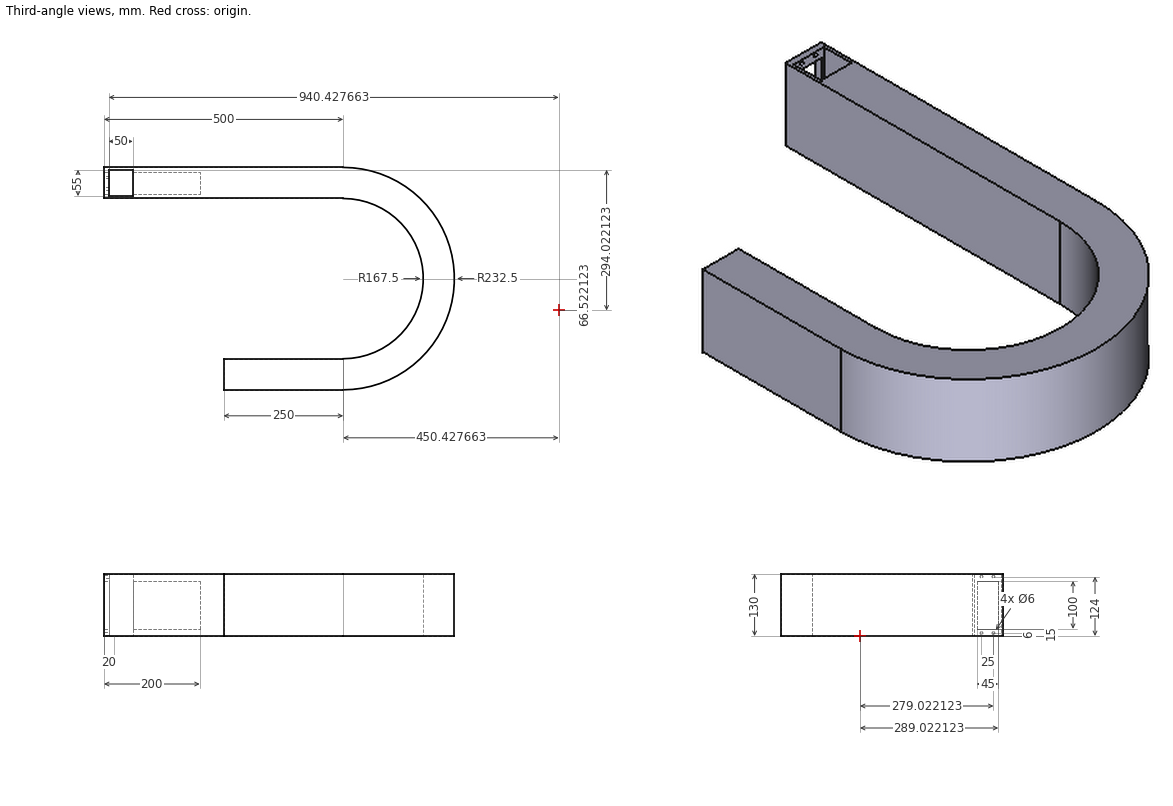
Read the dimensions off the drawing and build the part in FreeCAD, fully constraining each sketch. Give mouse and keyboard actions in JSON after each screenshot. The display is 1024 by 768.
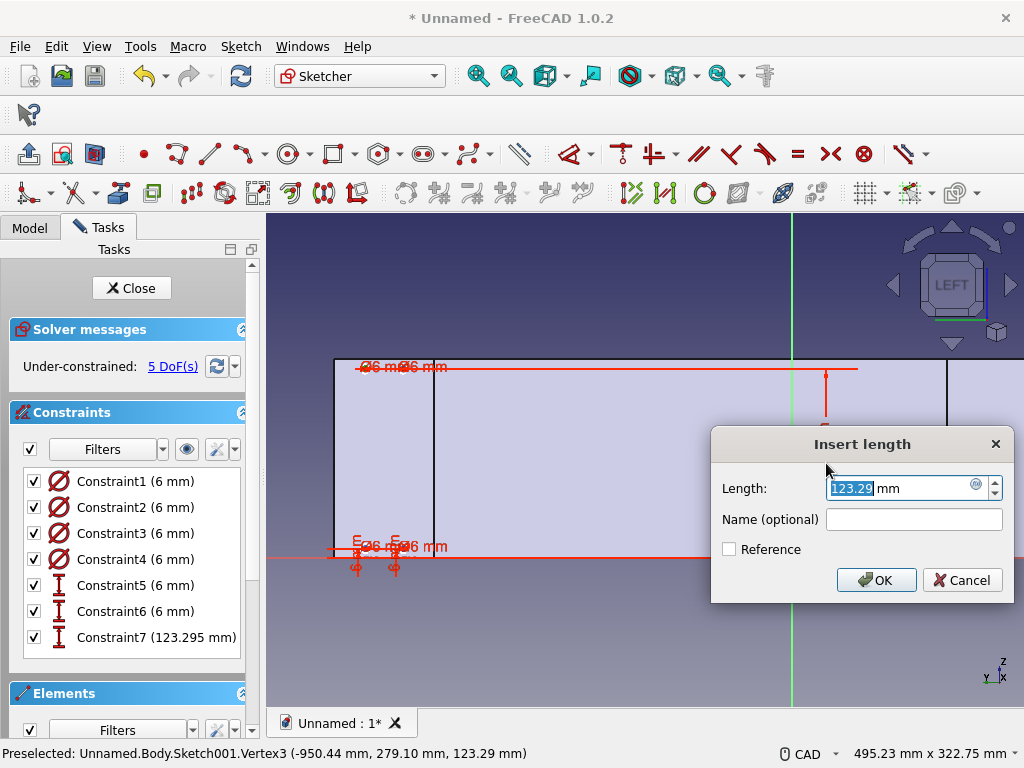
{"action": "type", "text": "124"}
{"action": "key", "text": "Return"}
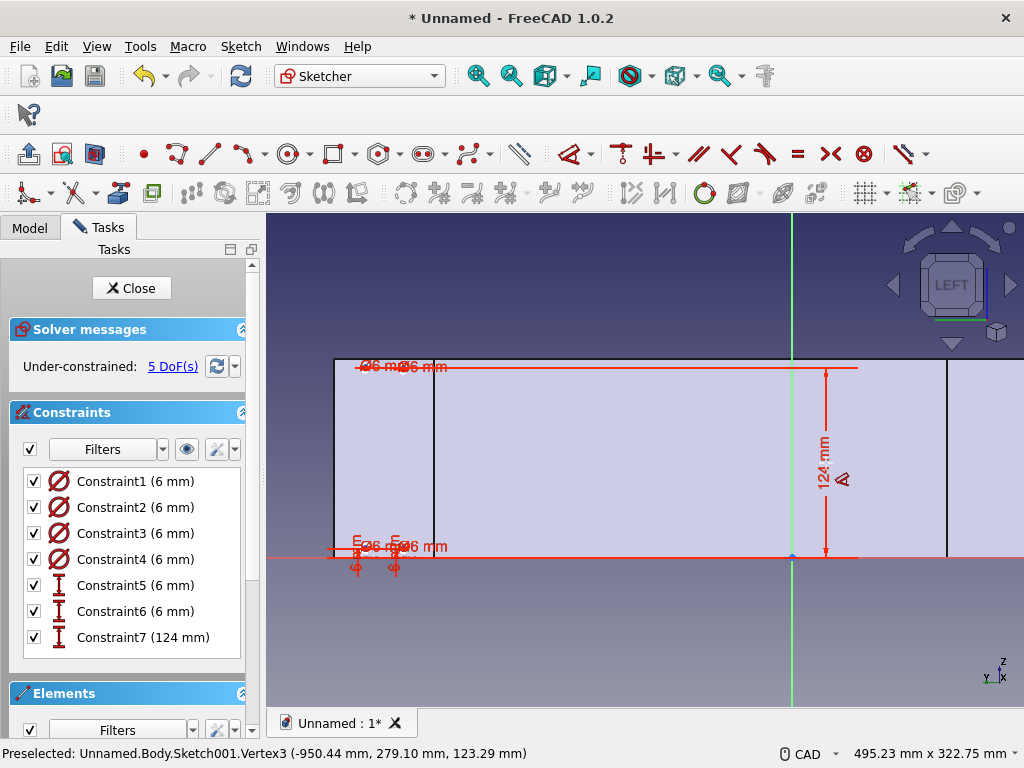
{"action": "left_click", "coordinate": [403, 369]}
{"action": "left_click", "coordinate": [826, 420]}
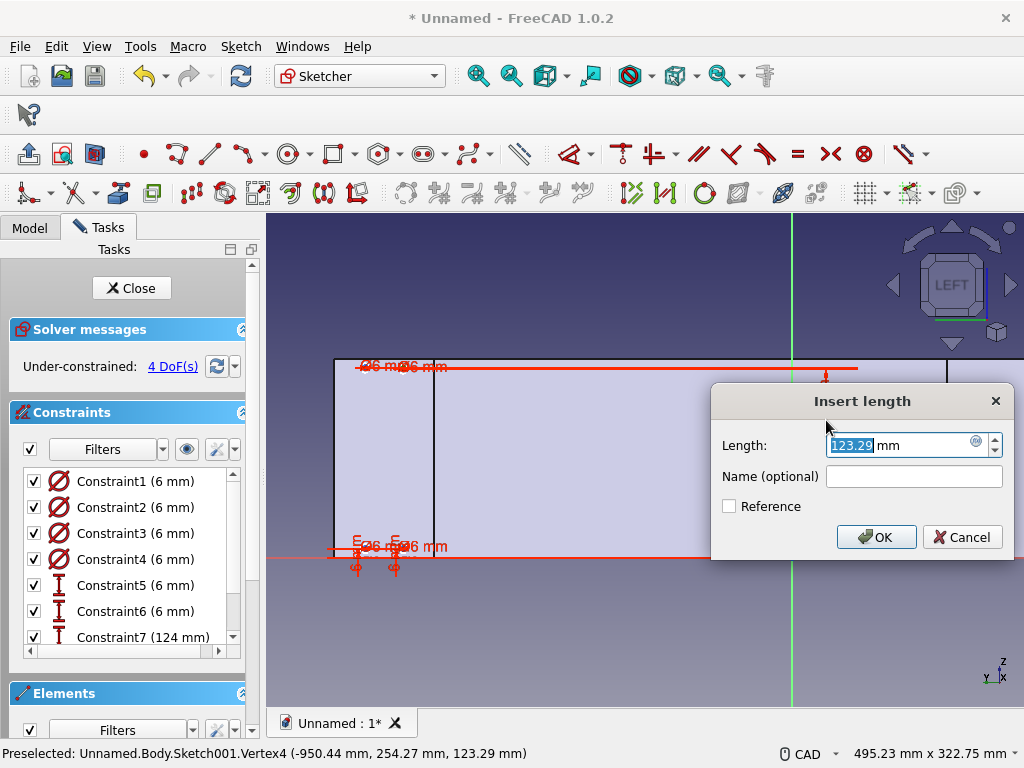
{"action": "type", "text": "124"}
{"action": "key", "text": "Return"}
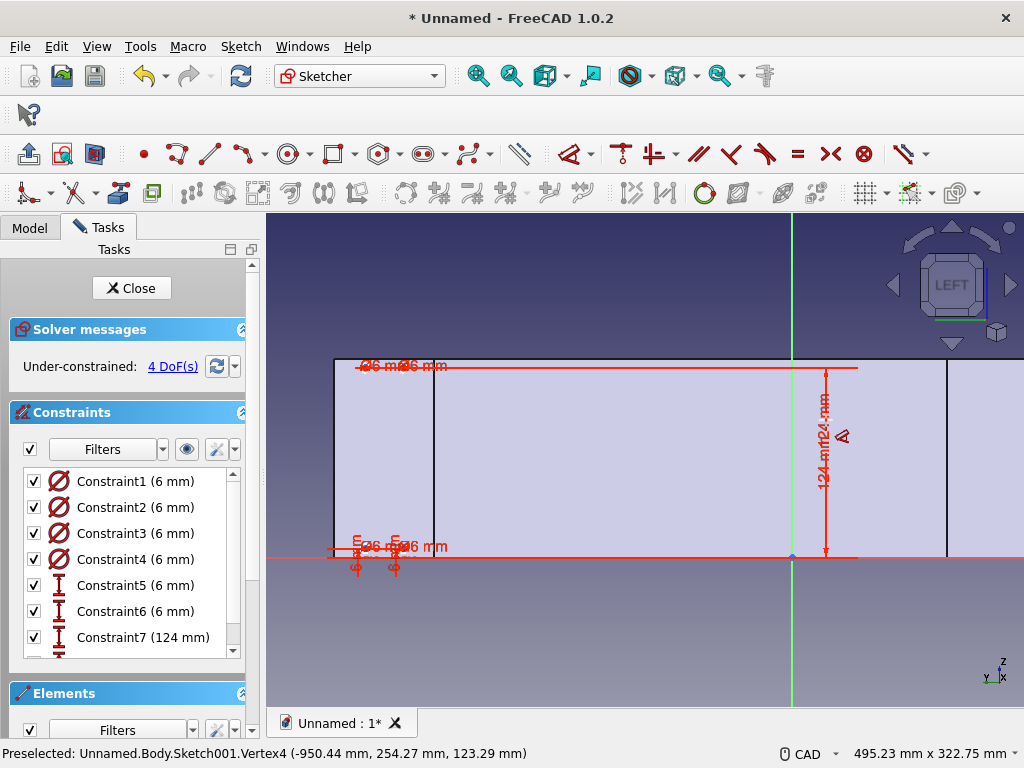
{"action": "left_click", "coordinate": [365, 549]}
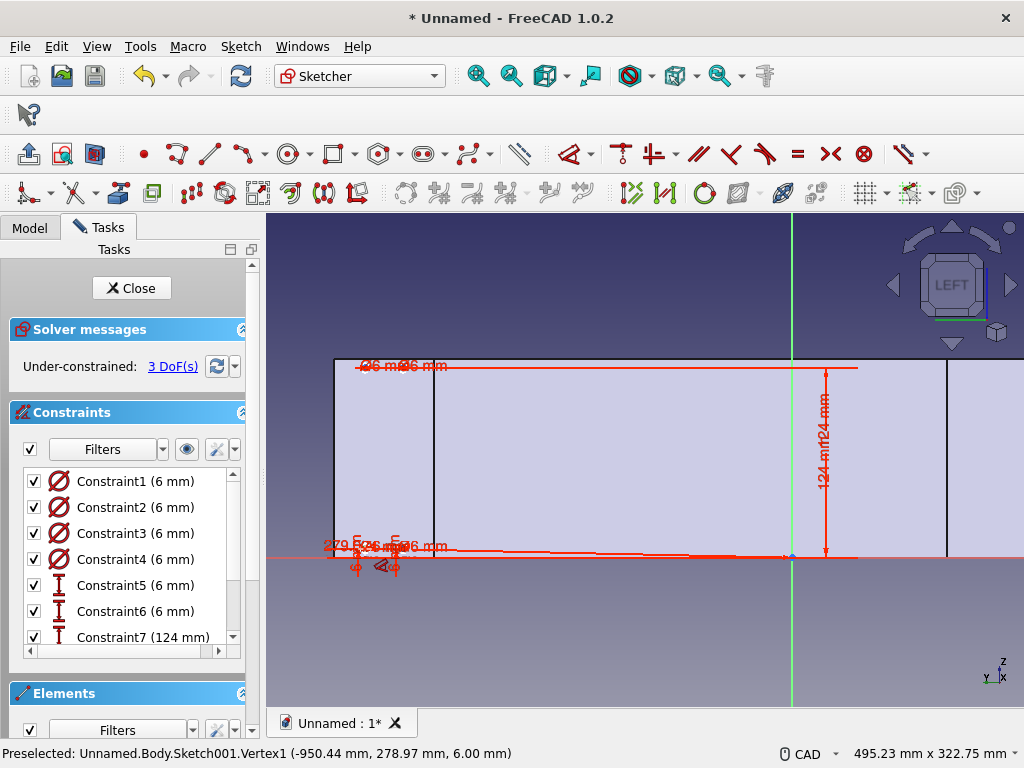
{"action": "left_click", "coordinate": [403, 549]}
{"action": "left_click", "coordinate": [384, 583]}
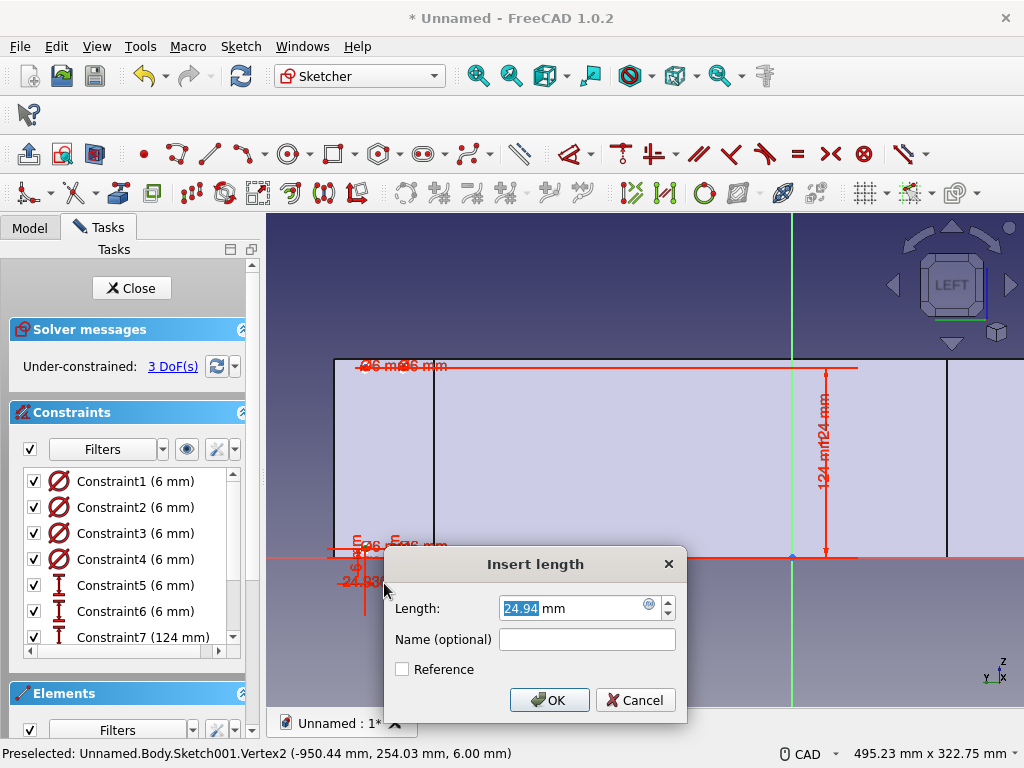
{"action": "type", "text": "25"}
{"action": "key", "text": "Return"}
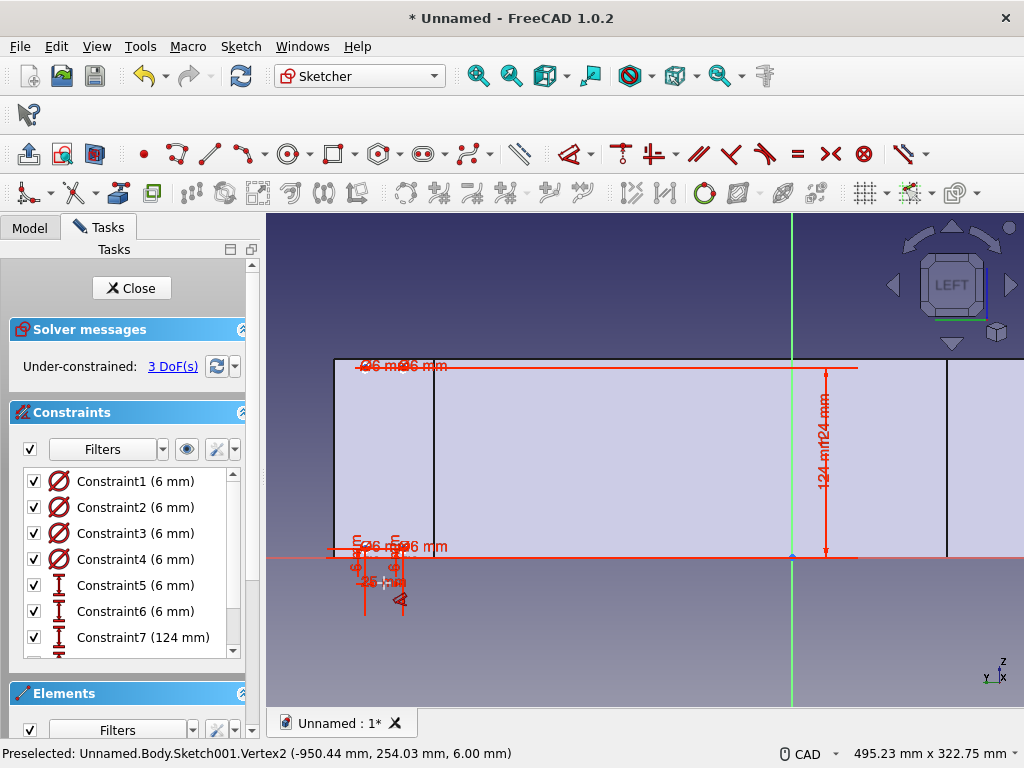
{"action": "left_click", "coordinate": [403, 549]}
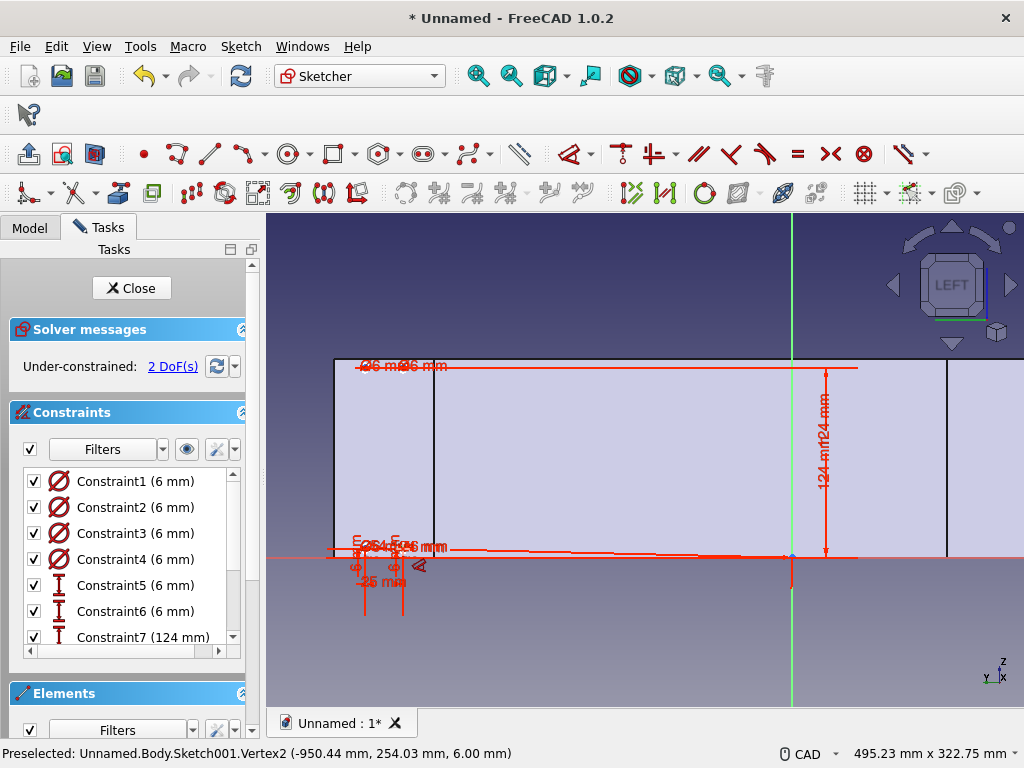
{"action": "left_click", "coordinate": [365, 368]}
{"action": "left_click", "coordinate": [384, 334]}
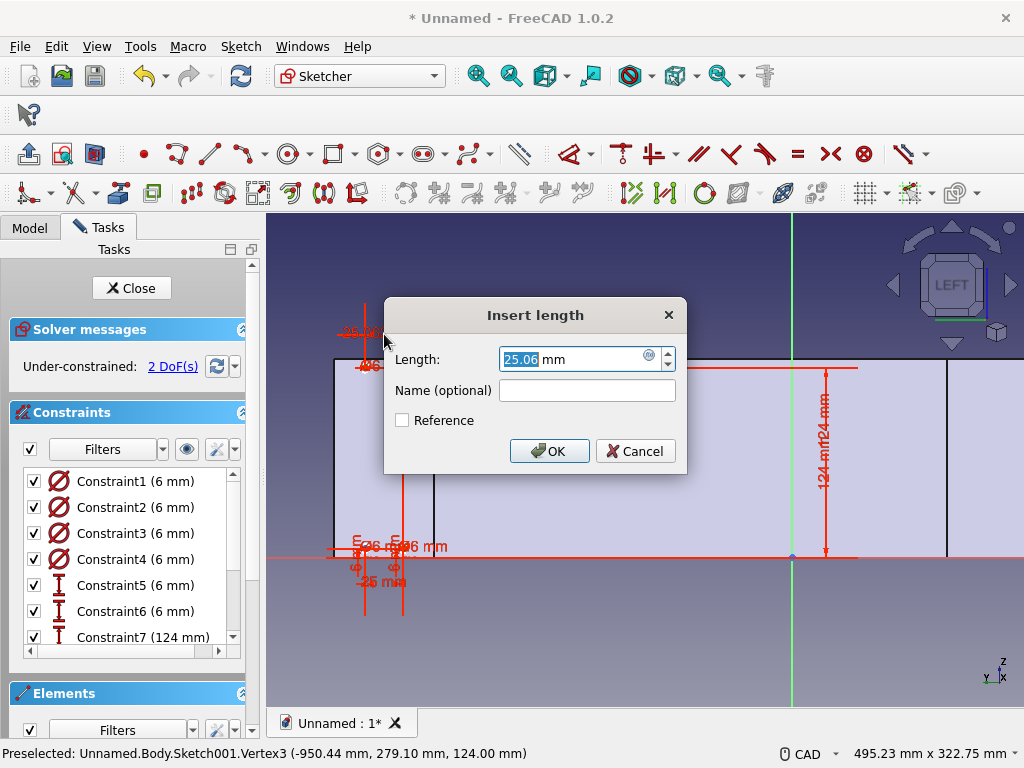
{"action": "type", "text": "25"}
{"action": "key", "text": "Return"}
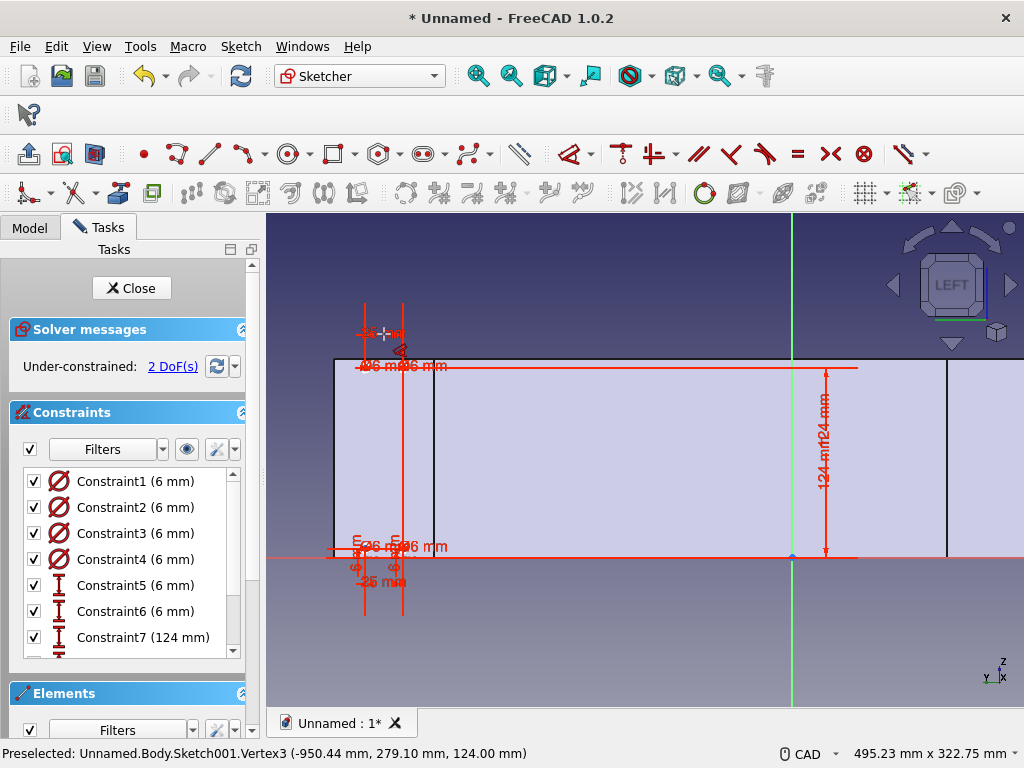
{"action": "left_click", "coordinate": [365, 368]}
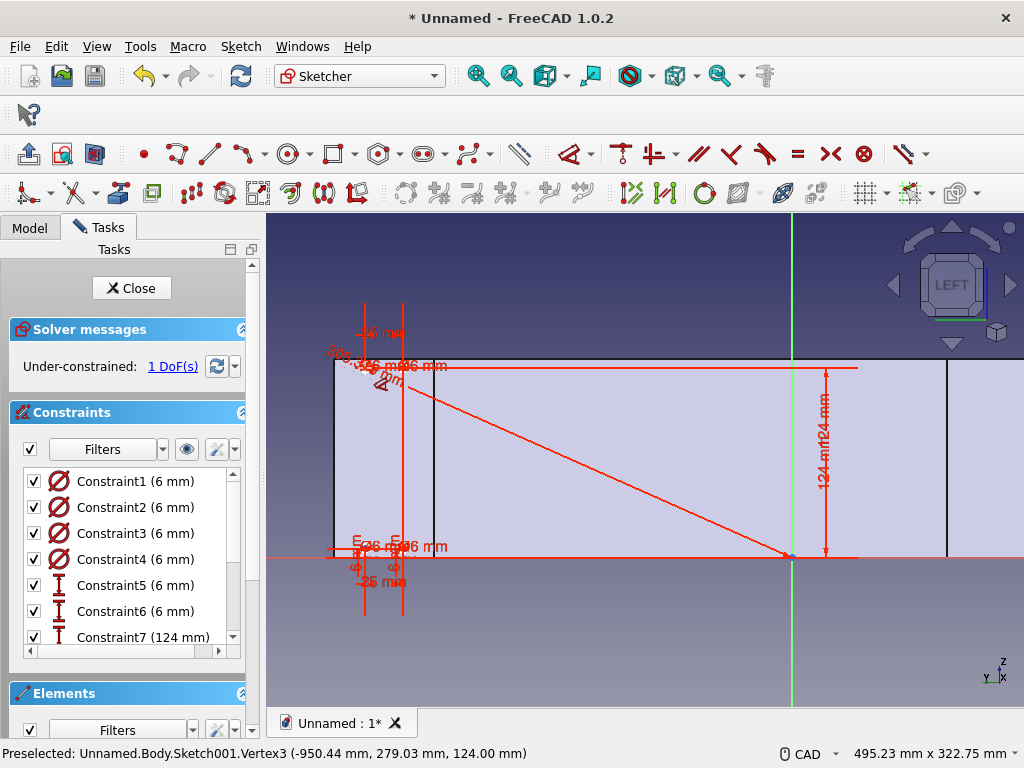
{"action": "left_click", "coordinate": [403, 368]}
{"action": "left_click", "coordinate": [384, 402]}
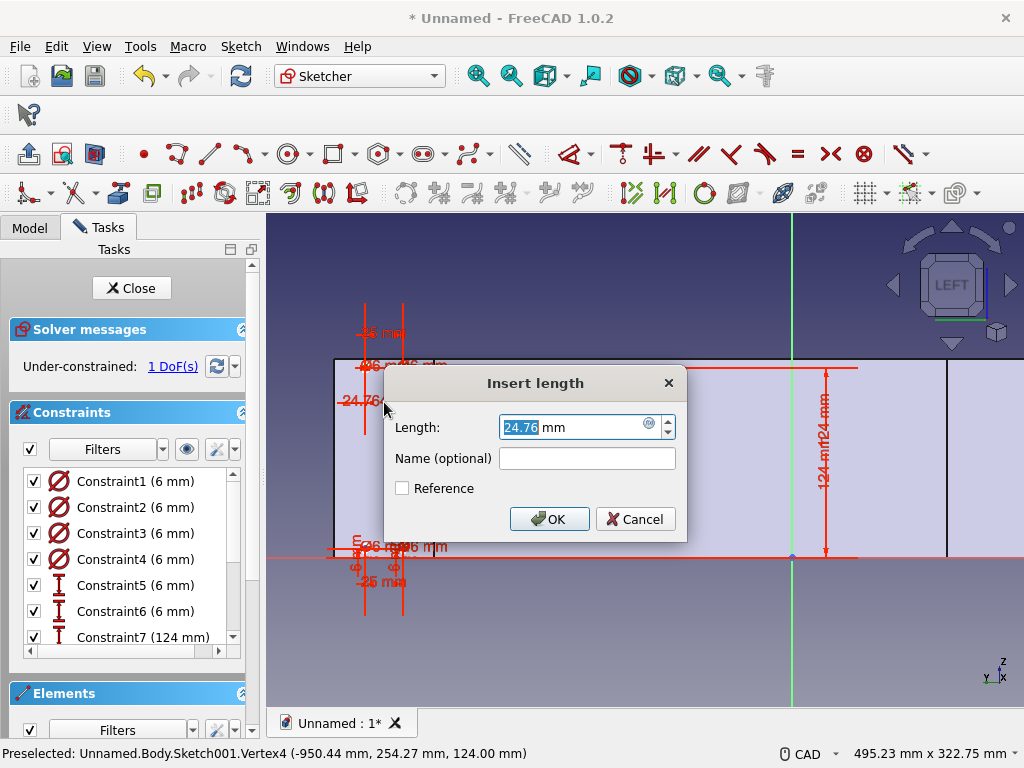
{"action": "type", "text": "25"}
{"action": "key", "text": "Return"}